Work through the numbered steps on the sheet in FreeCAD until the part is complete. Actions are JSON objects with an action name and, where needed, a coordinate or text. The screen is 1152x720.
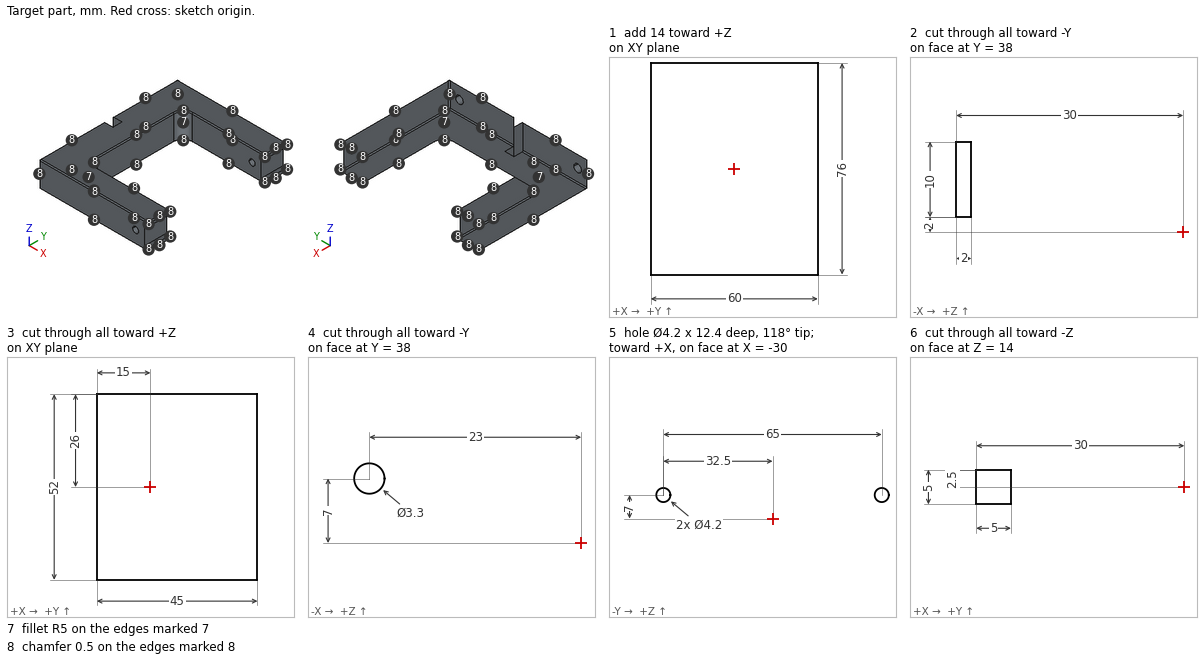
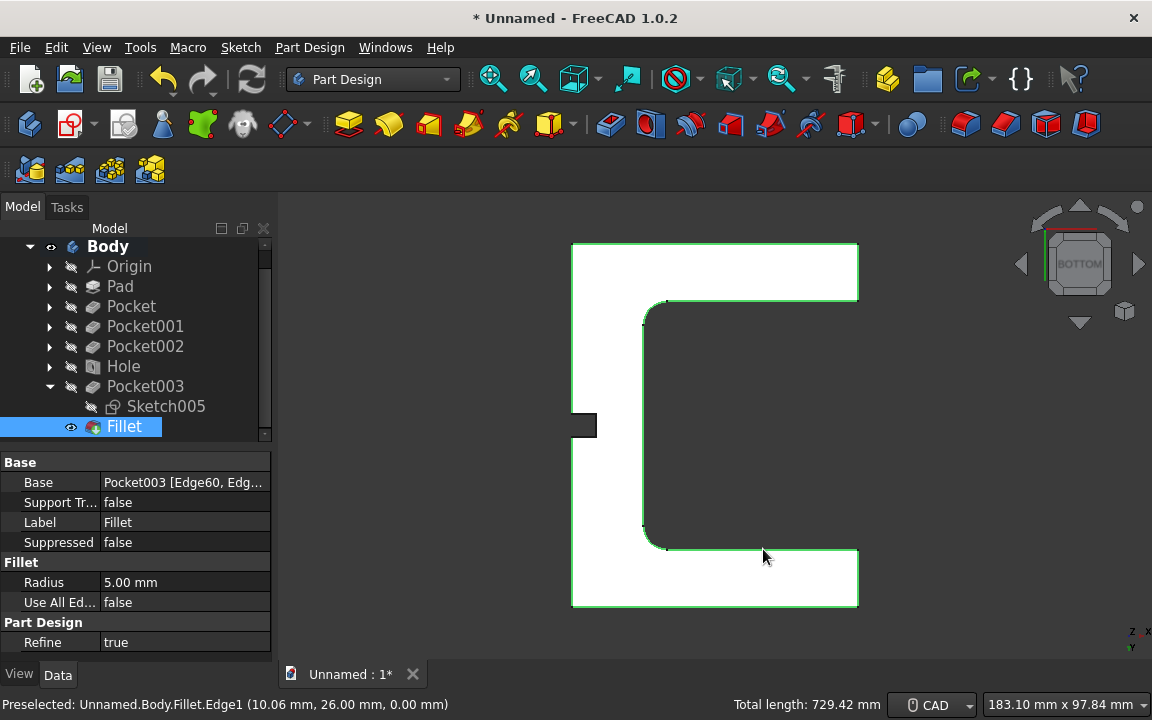
{"action": "scroll", "coordinate": [858, 300], "scroll_direction": "up", "scroll_amount": 8}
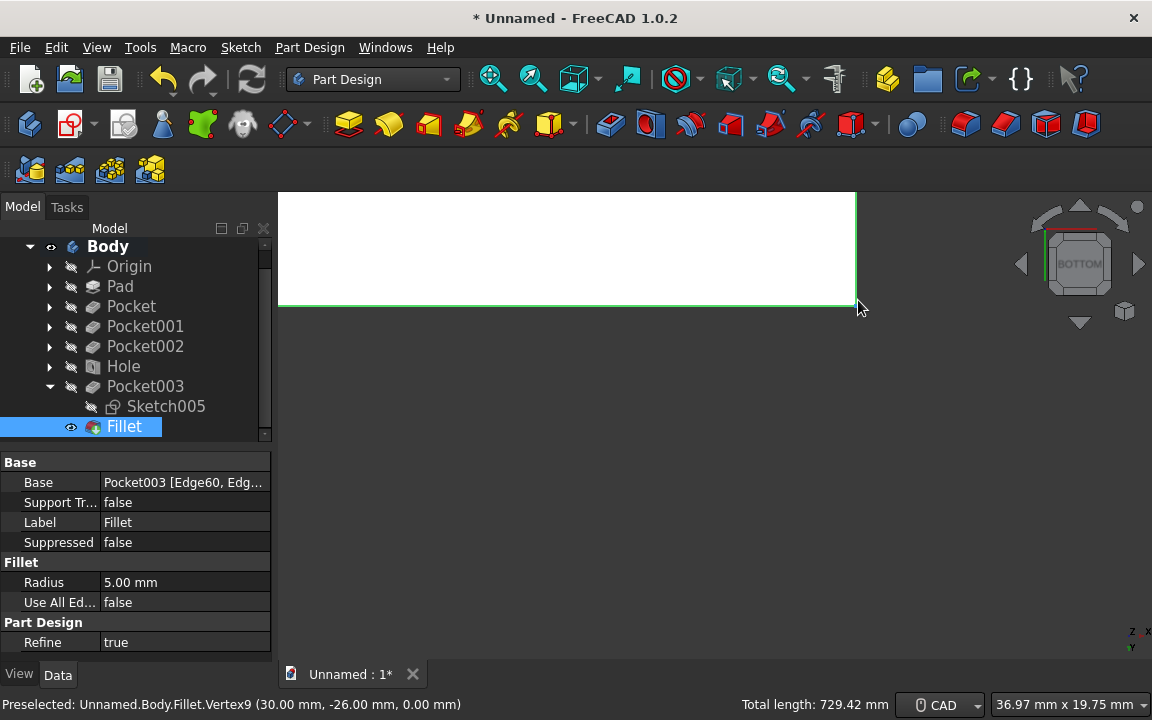
{"action": "key", "text": "v f"}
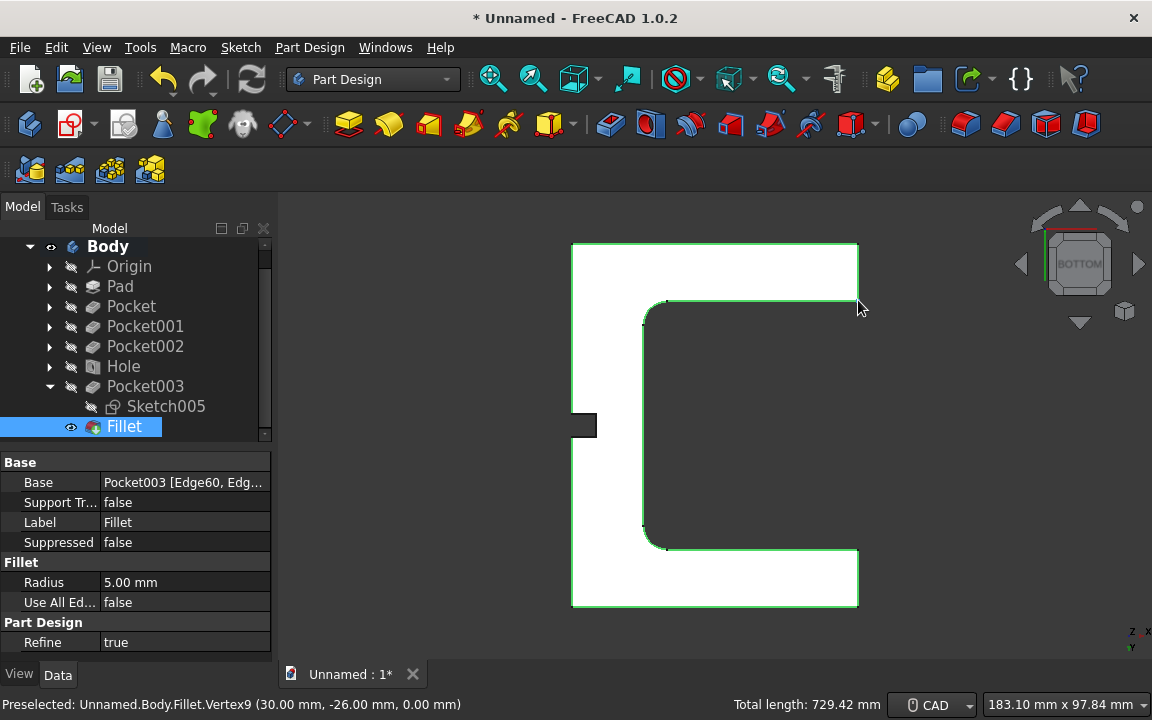
{"action": "key", "text": "4"}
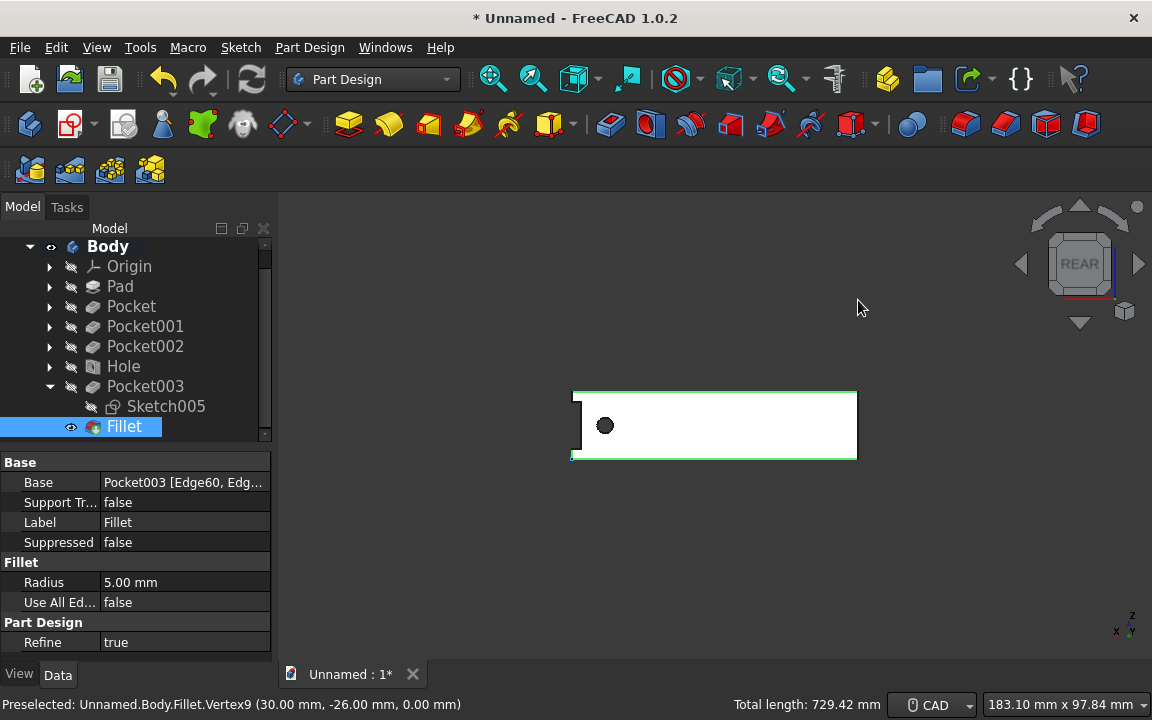
{"action": "key", "text": "v f"}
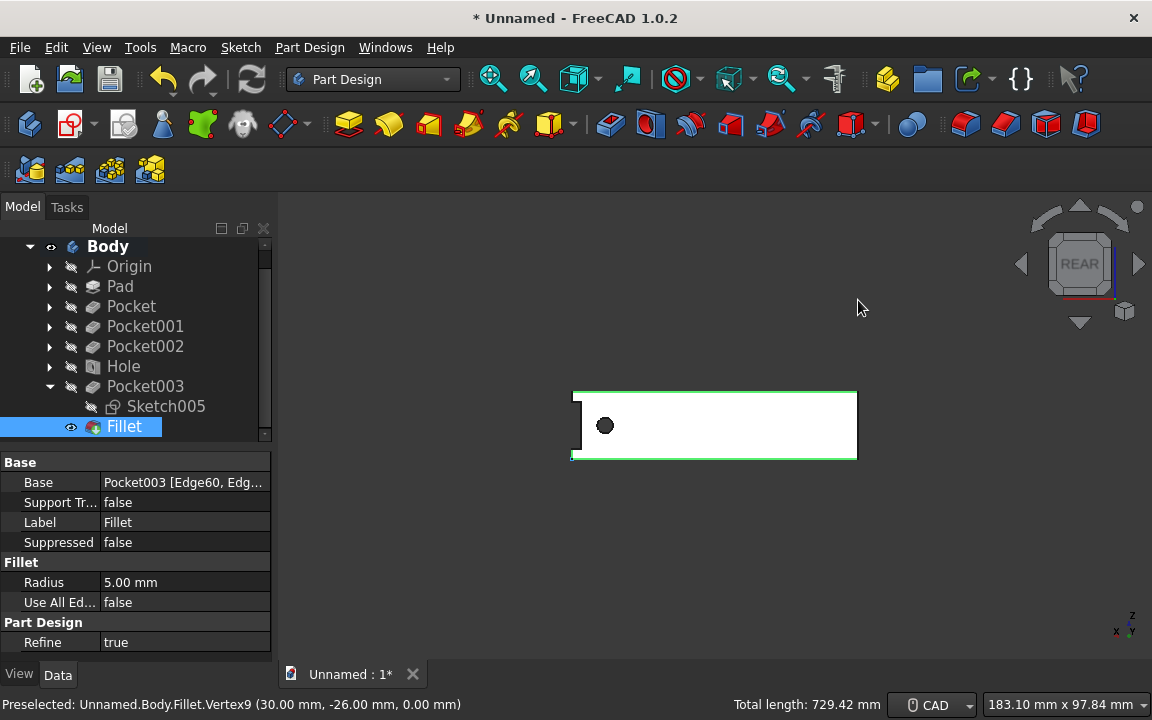
{"action": "left_click", "coordinate": [858, 425], "text": "ctrl"}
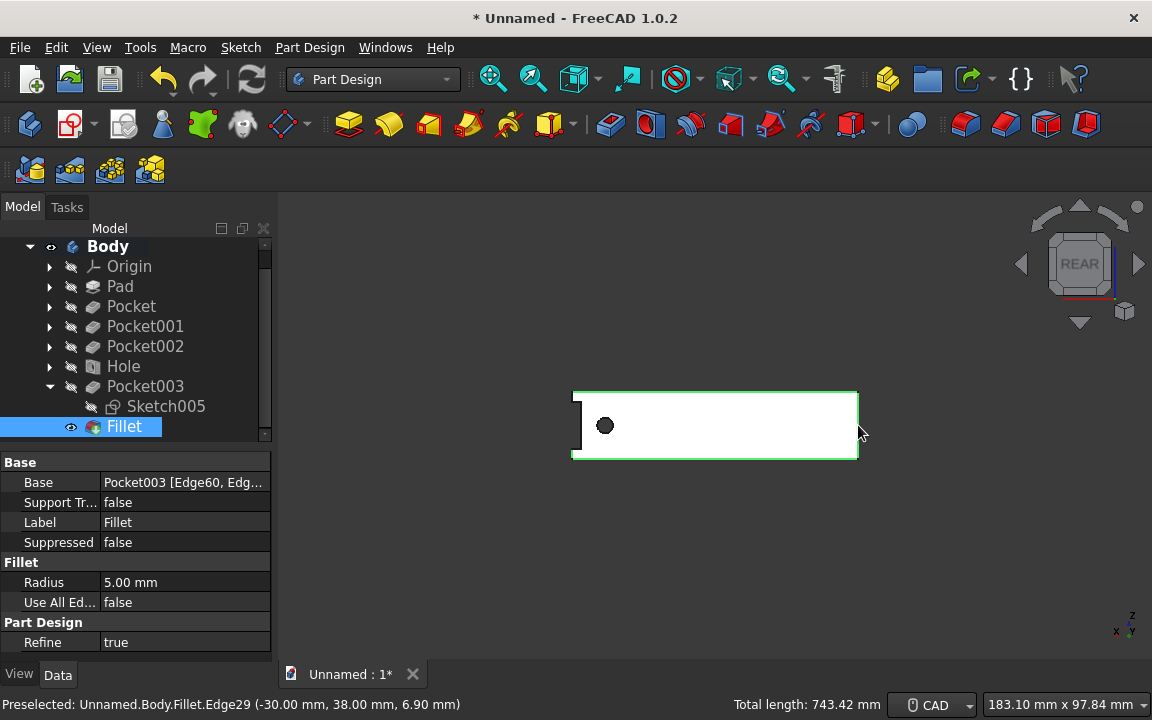
{"action": "scroll", "coordinate": [572, 396], "scroll_direction": "up", "scroll_amount": 8}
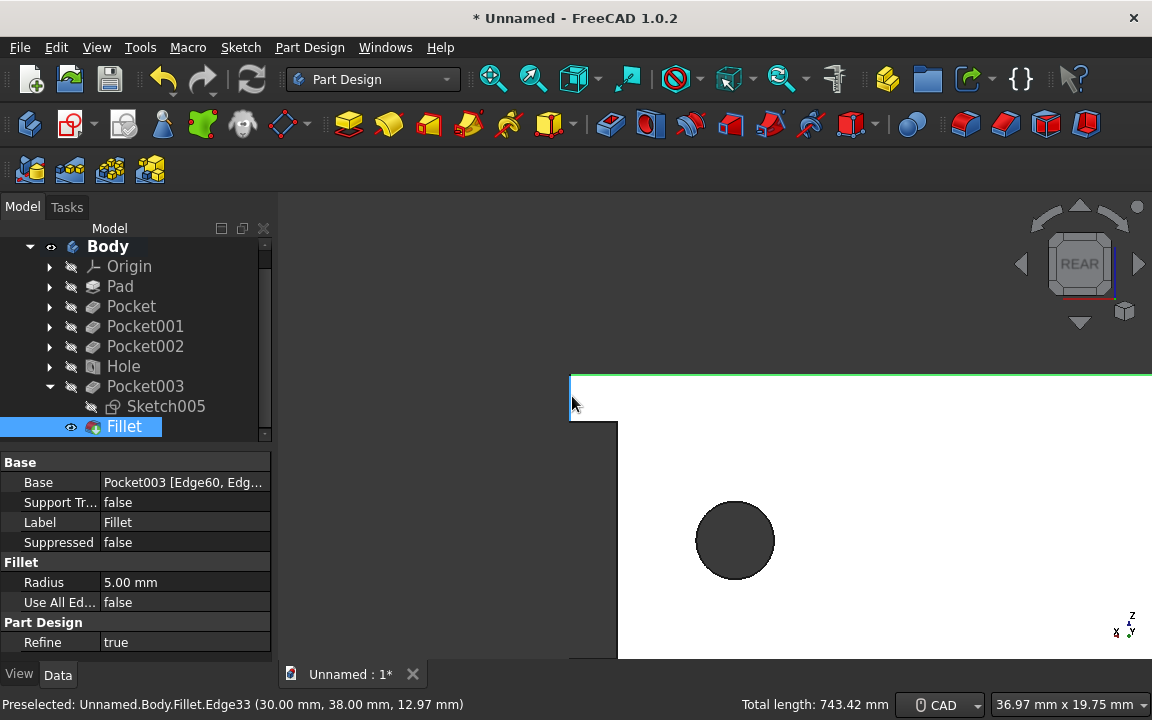
{"action": "left_click", "coordinate": [570, 398], "text": "ctrl"}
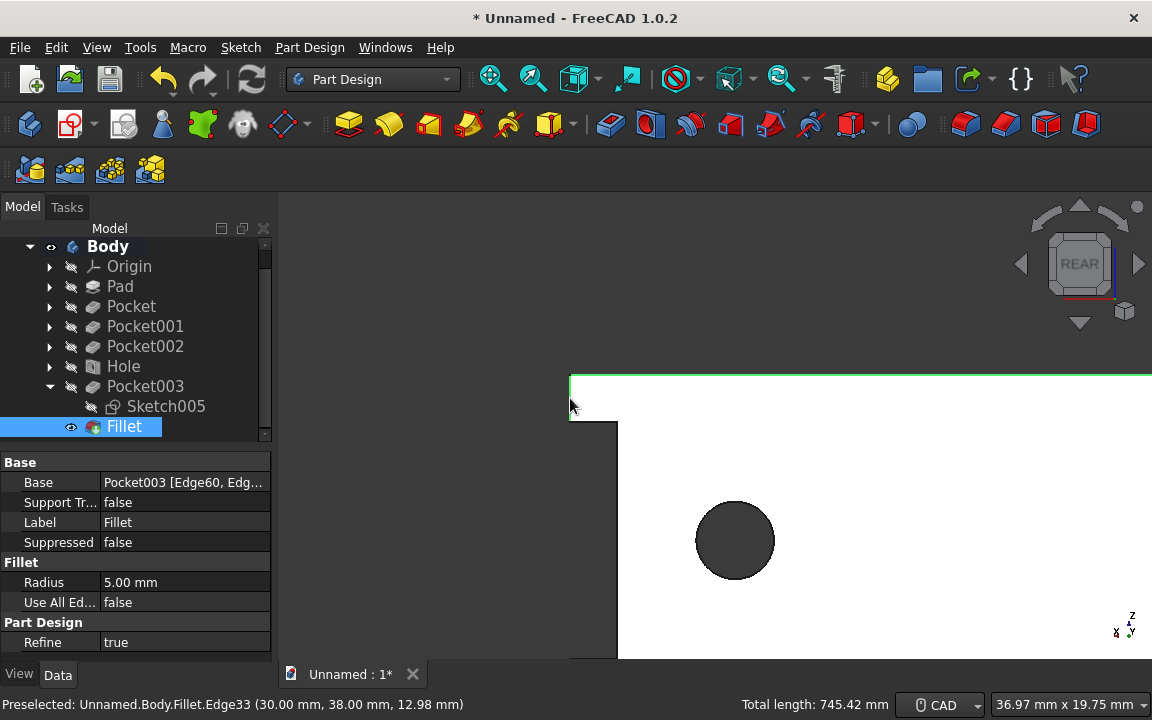
{"action": "key", "text": "v f"}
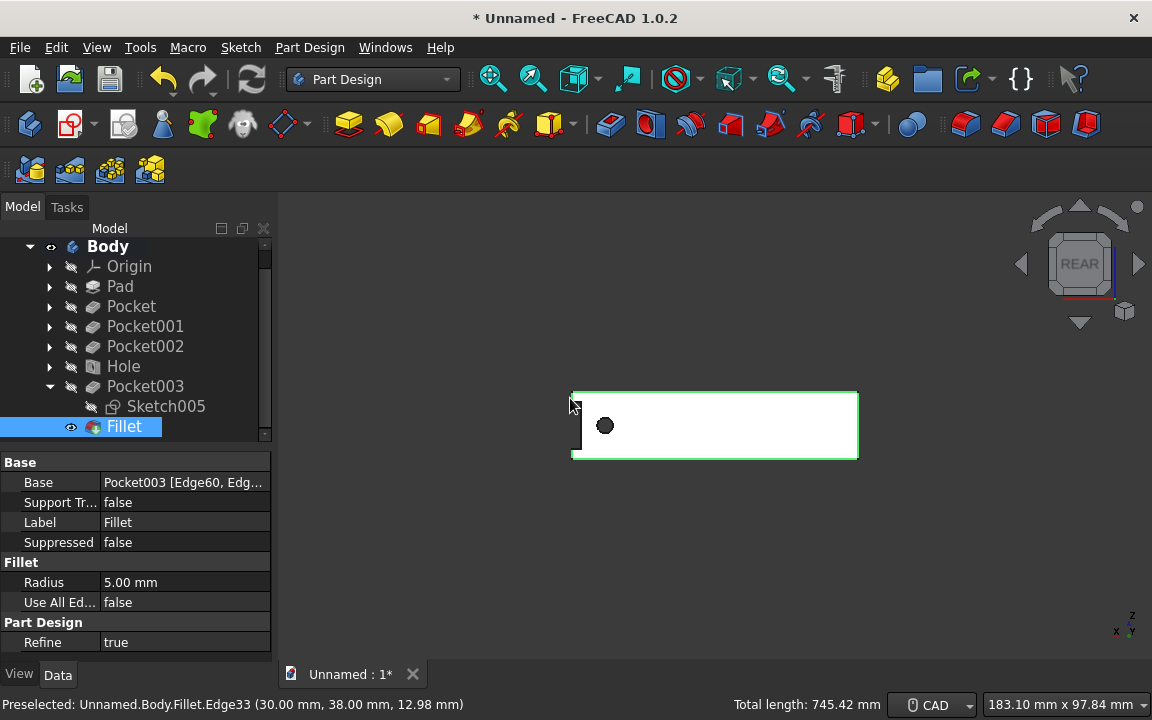
{"action": "key", "text": "6"}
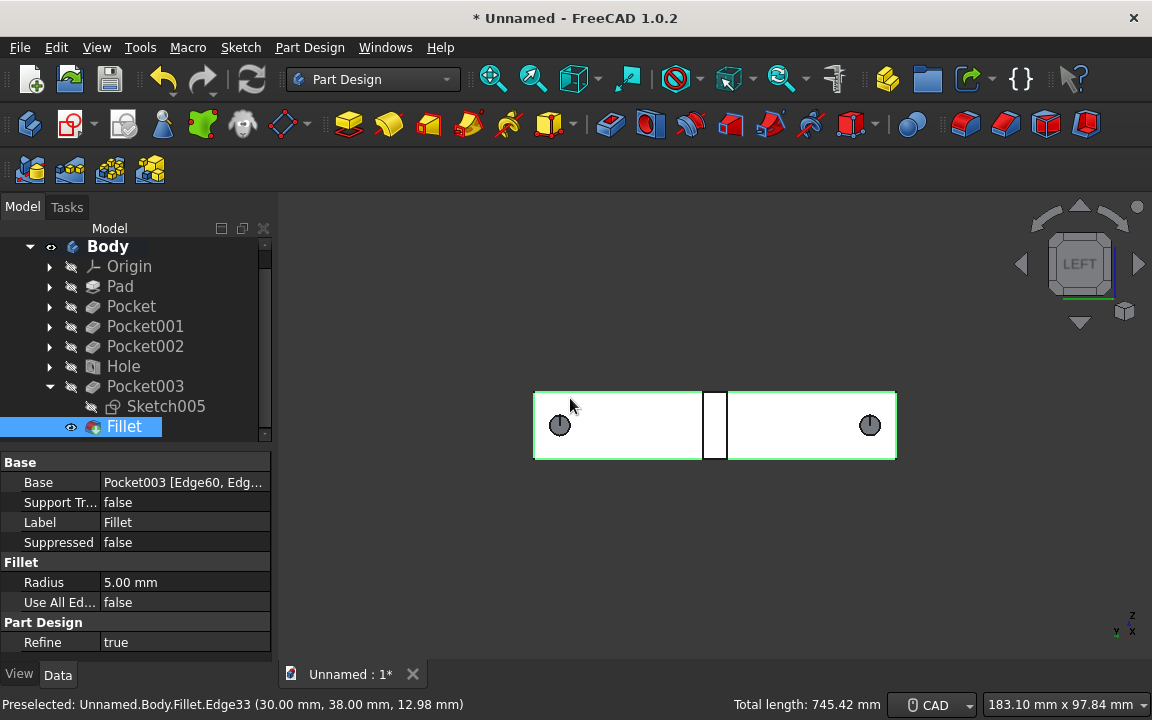
{"action": "left_click", "coordinate": [494, 80]}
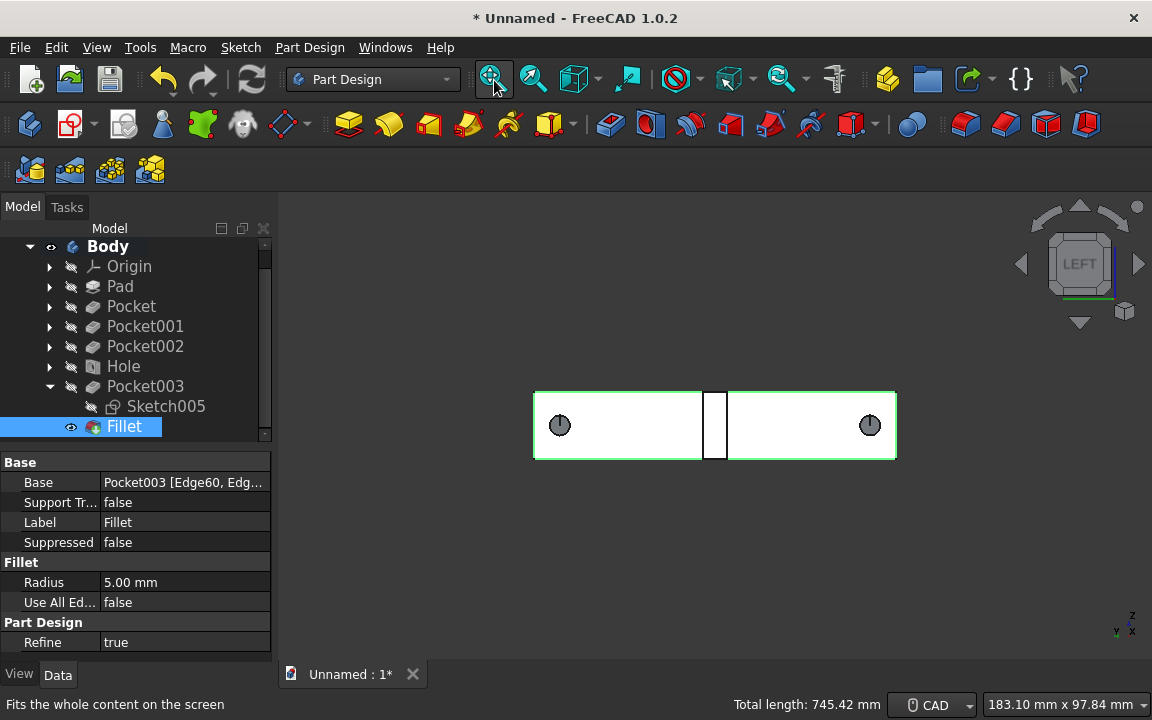
{"action": "scroll", "coordinate": [839, 396], "scroll_direction": "up", "scroll_amount": 8}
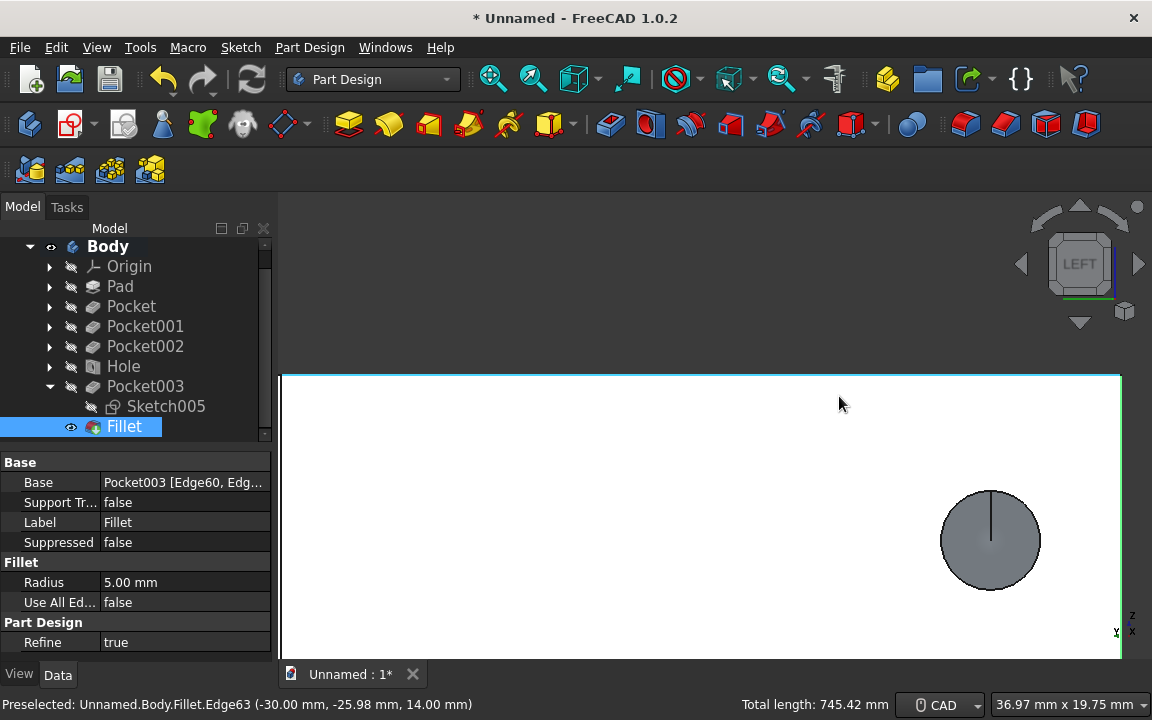
{"action": "left_click", "coordinate": [494, 80]}